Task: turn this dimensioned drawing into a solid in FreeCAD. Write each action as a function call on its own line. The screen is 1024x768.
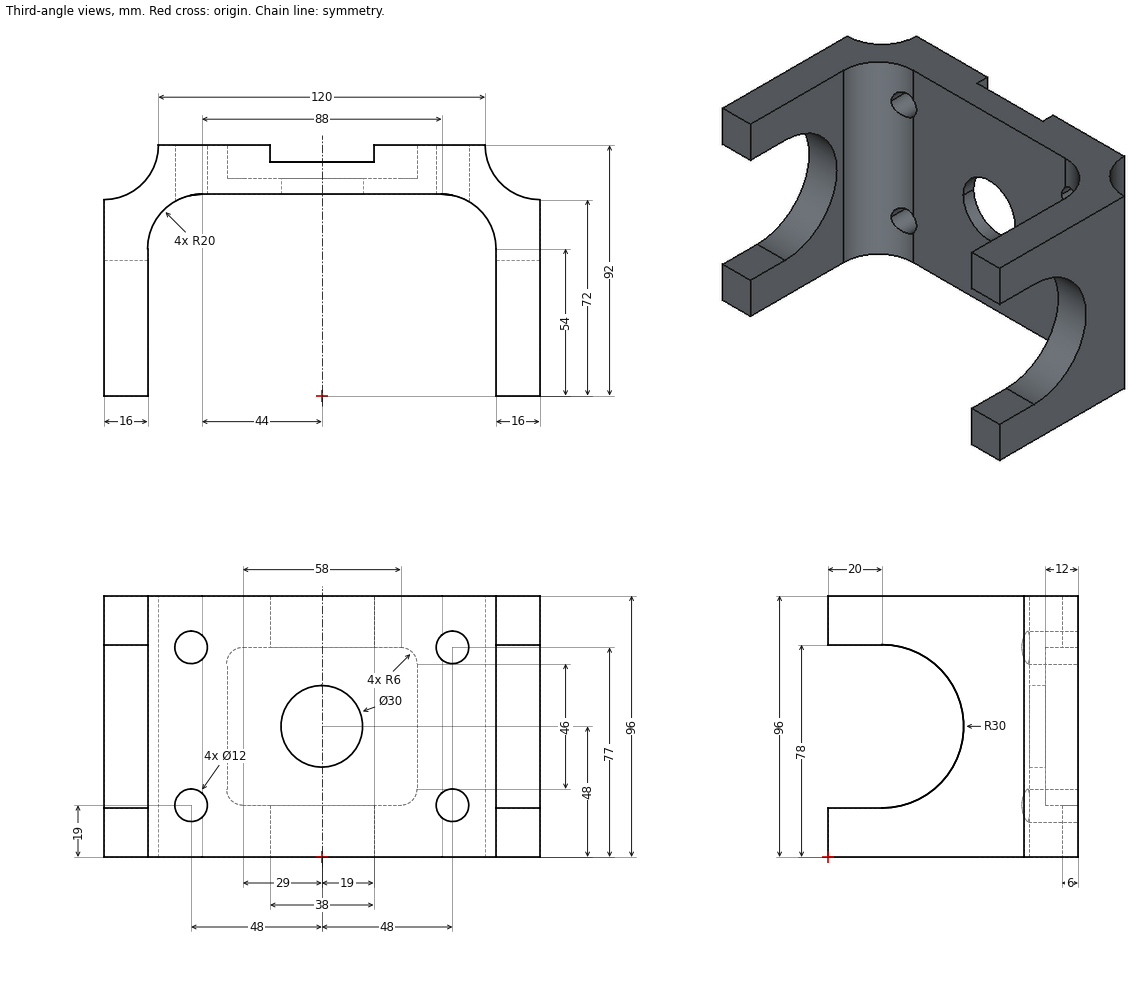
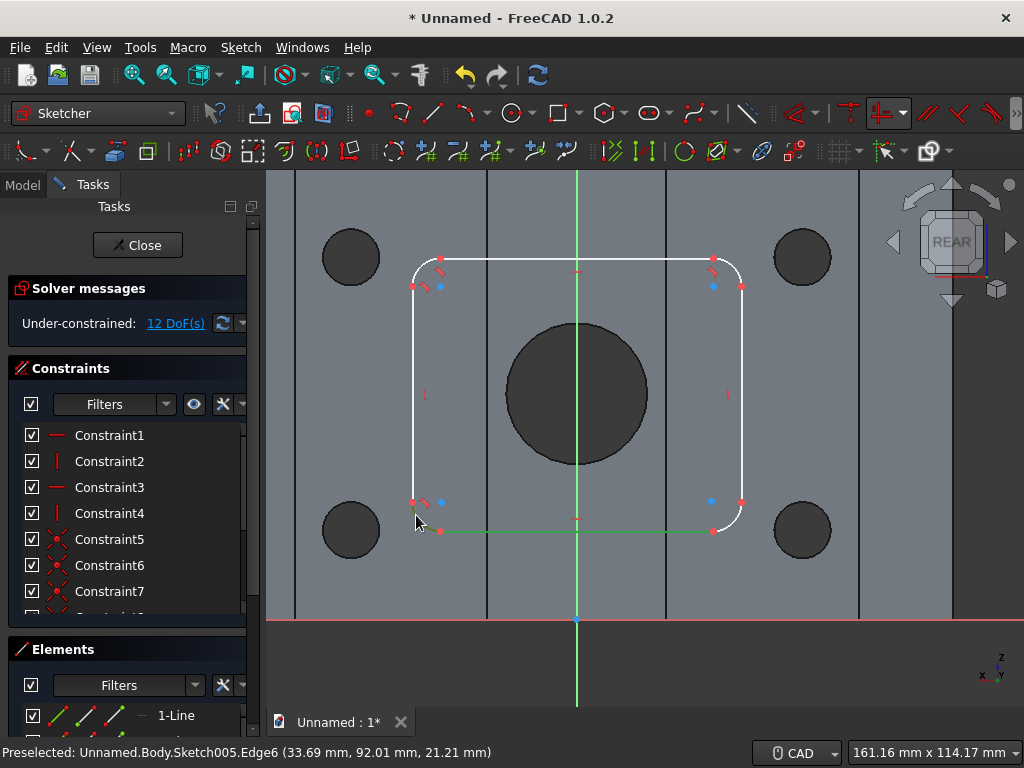
click(992, 114)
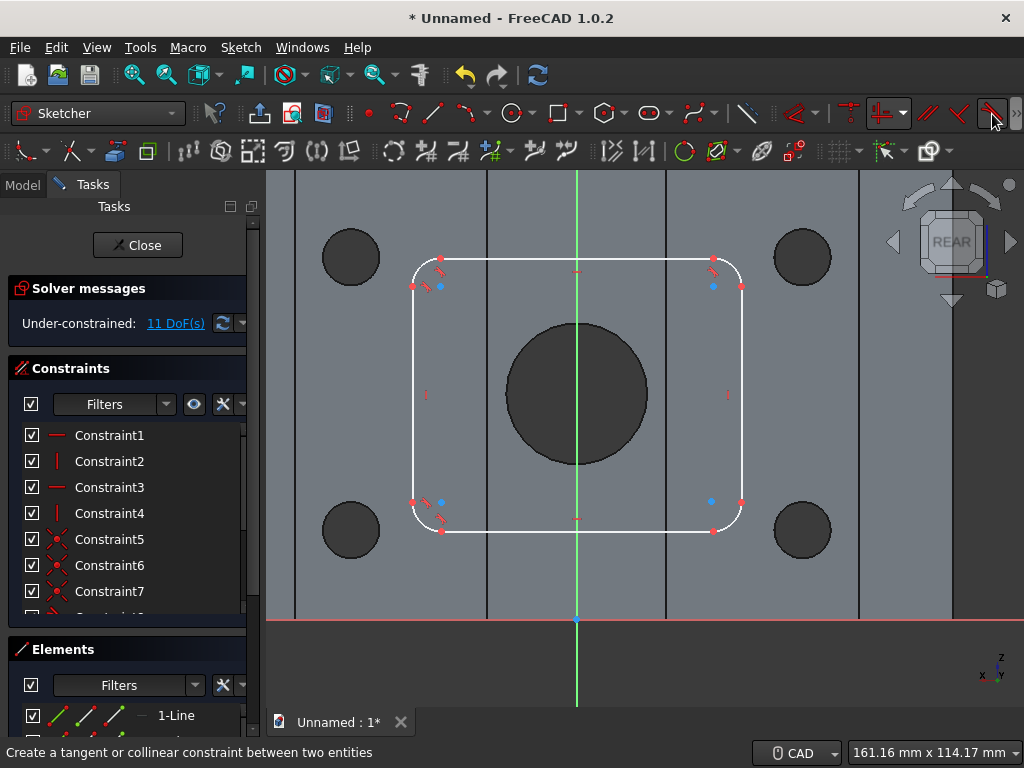
click(523, 532)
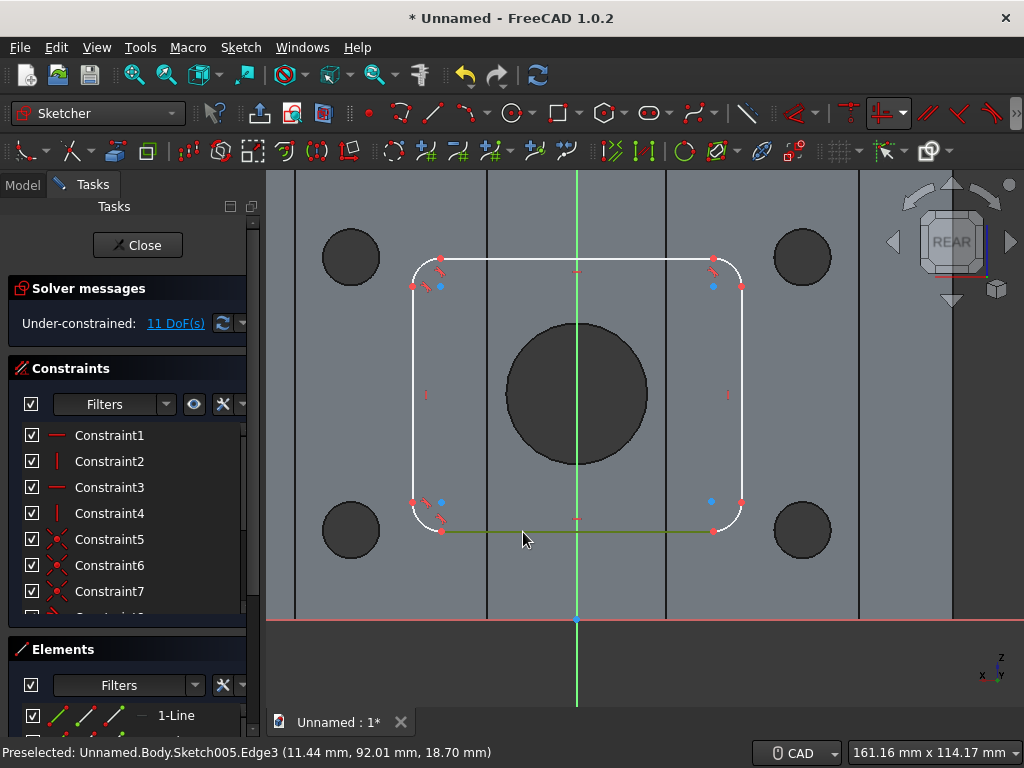
click(726, 528)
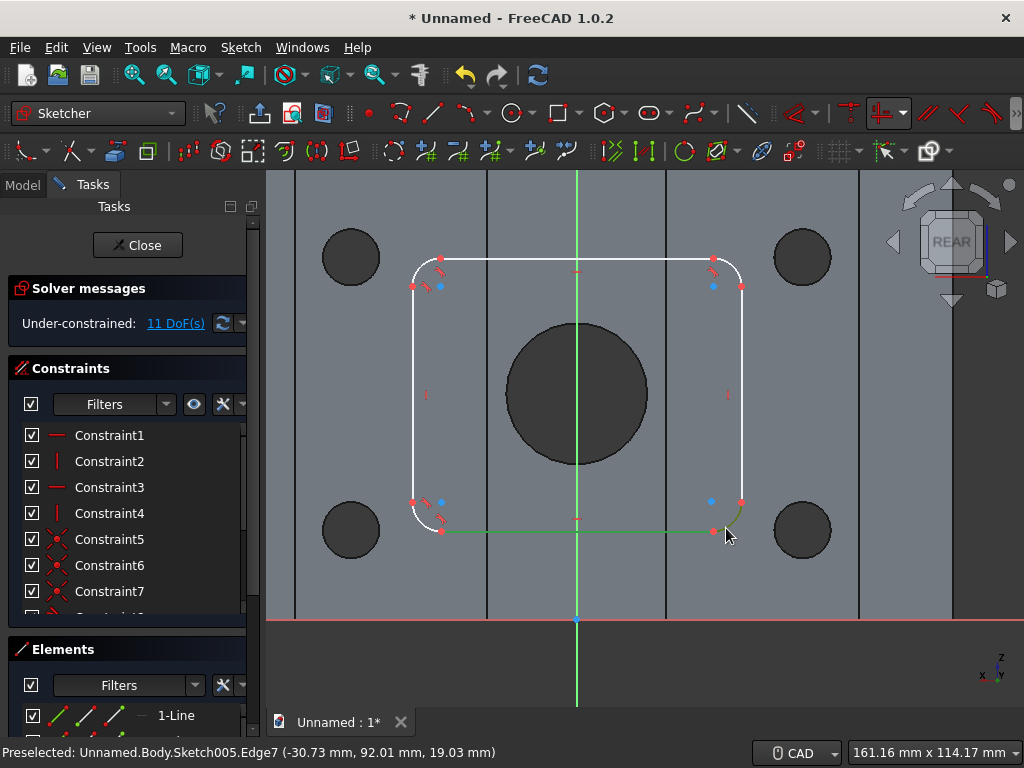
click(992, 114)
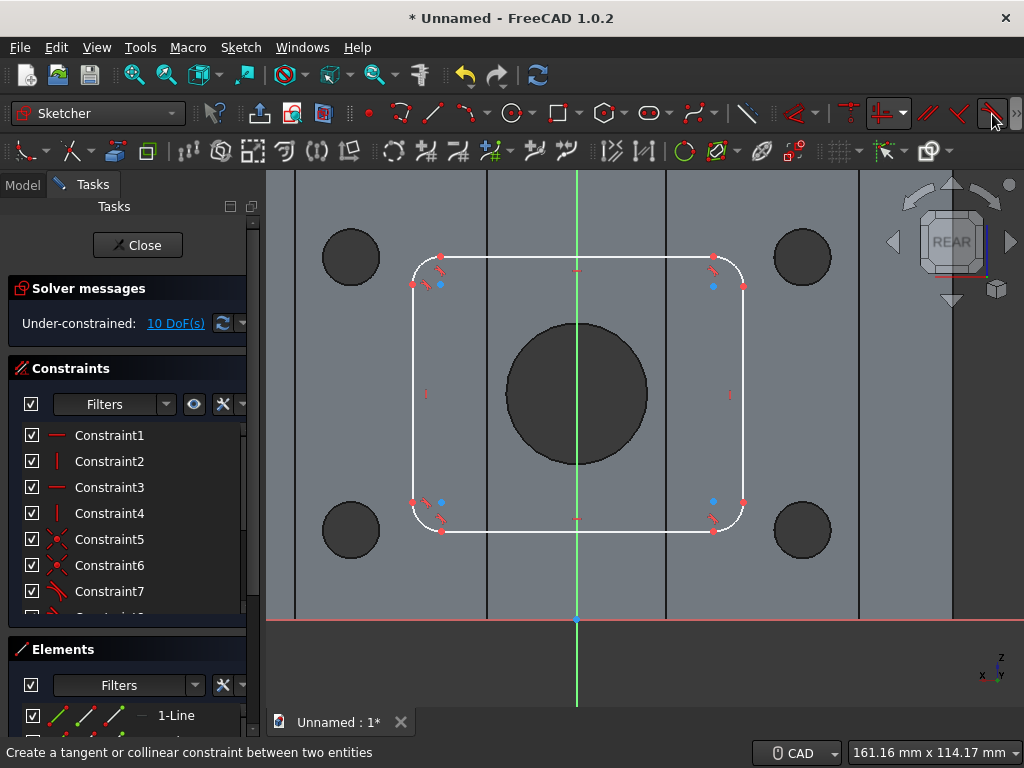
click(743, 438)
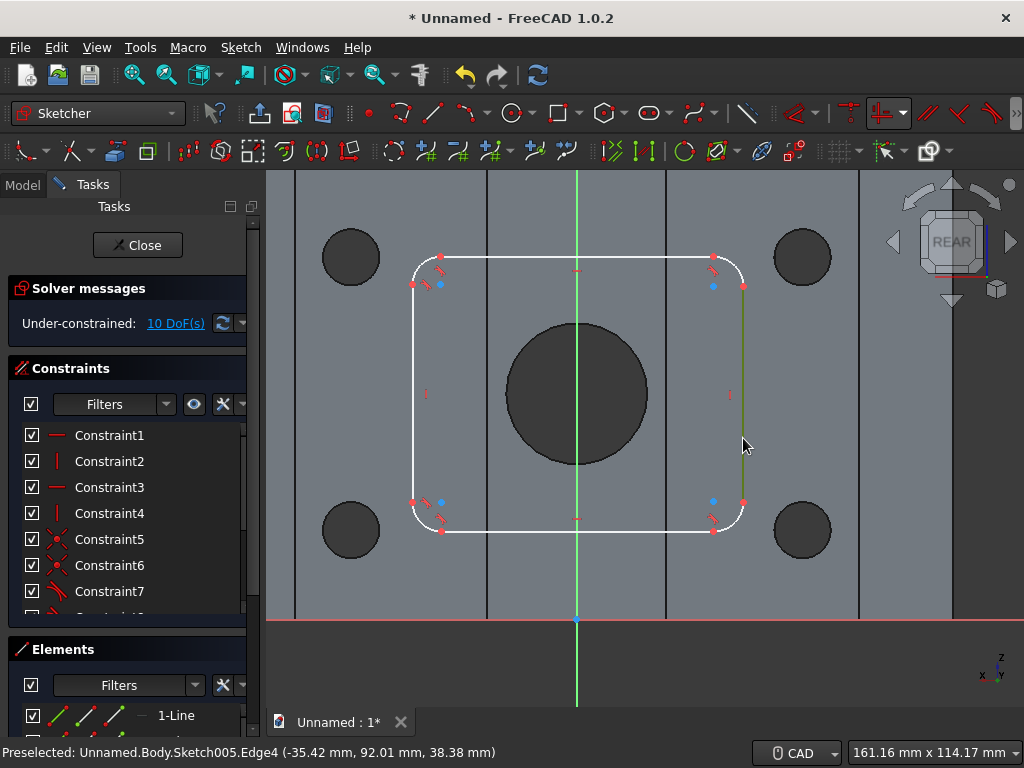
click(727, 528)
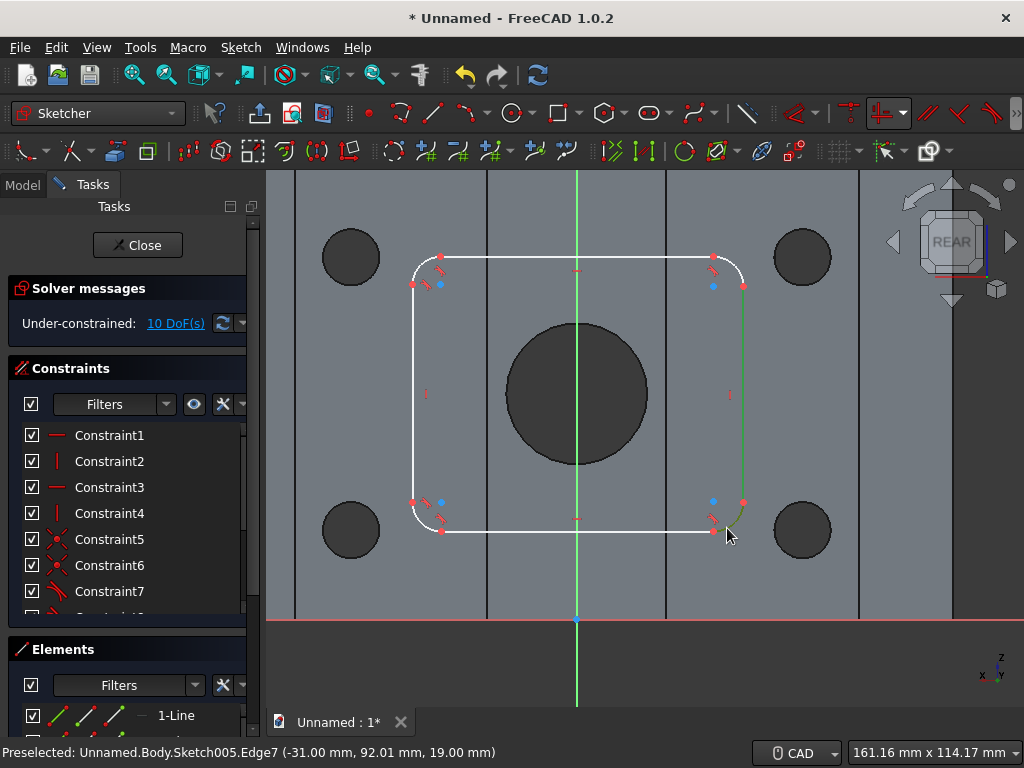
click(992, 114)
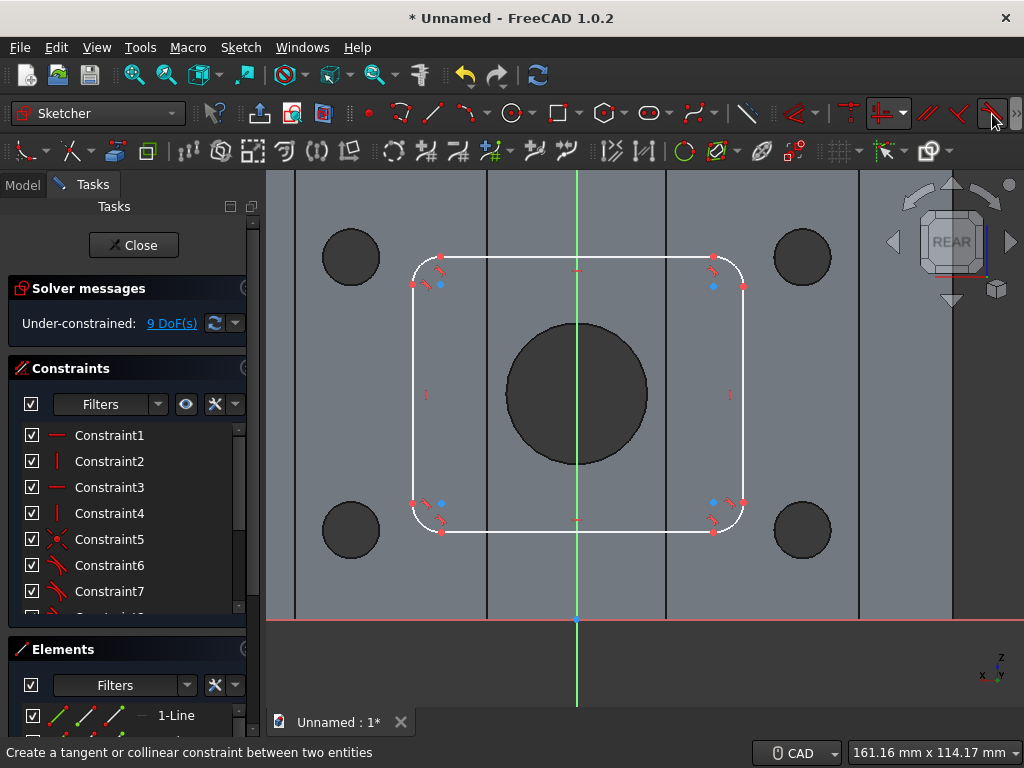
click(743, 438)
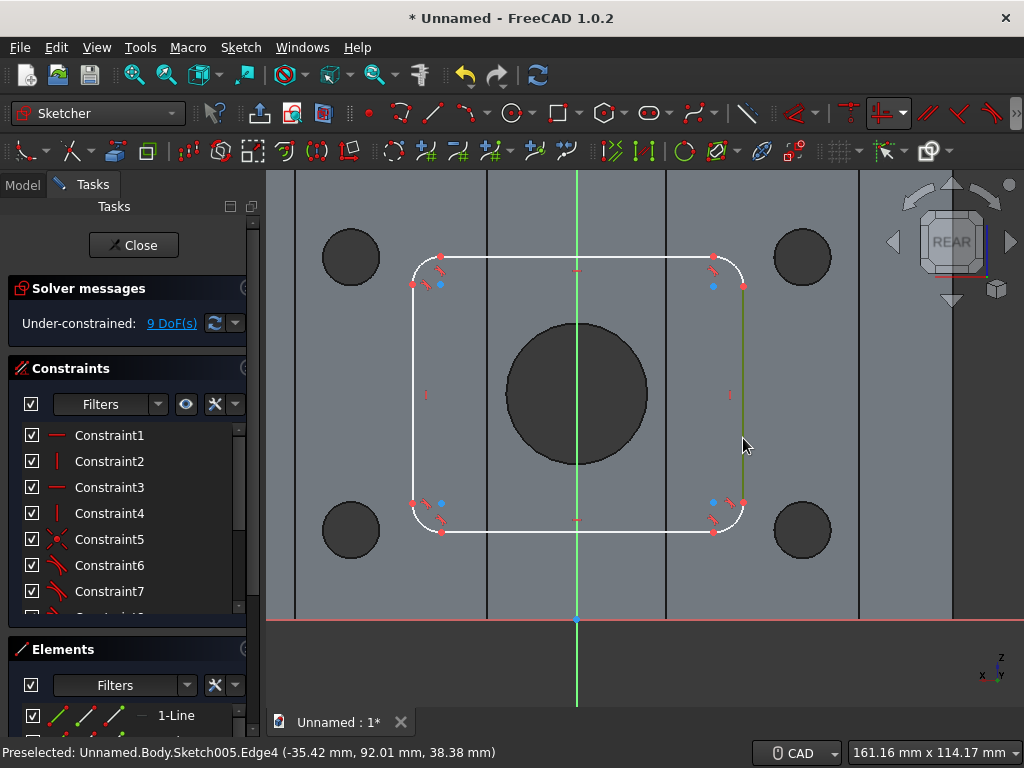
click(740, 273)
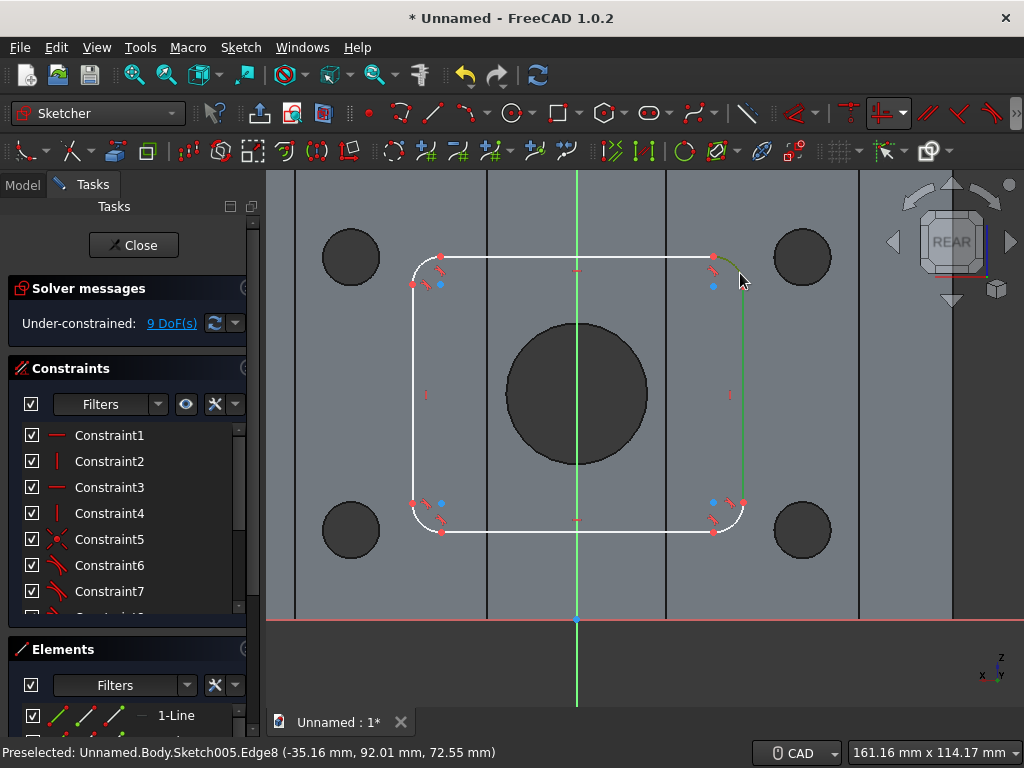
click(992, 114)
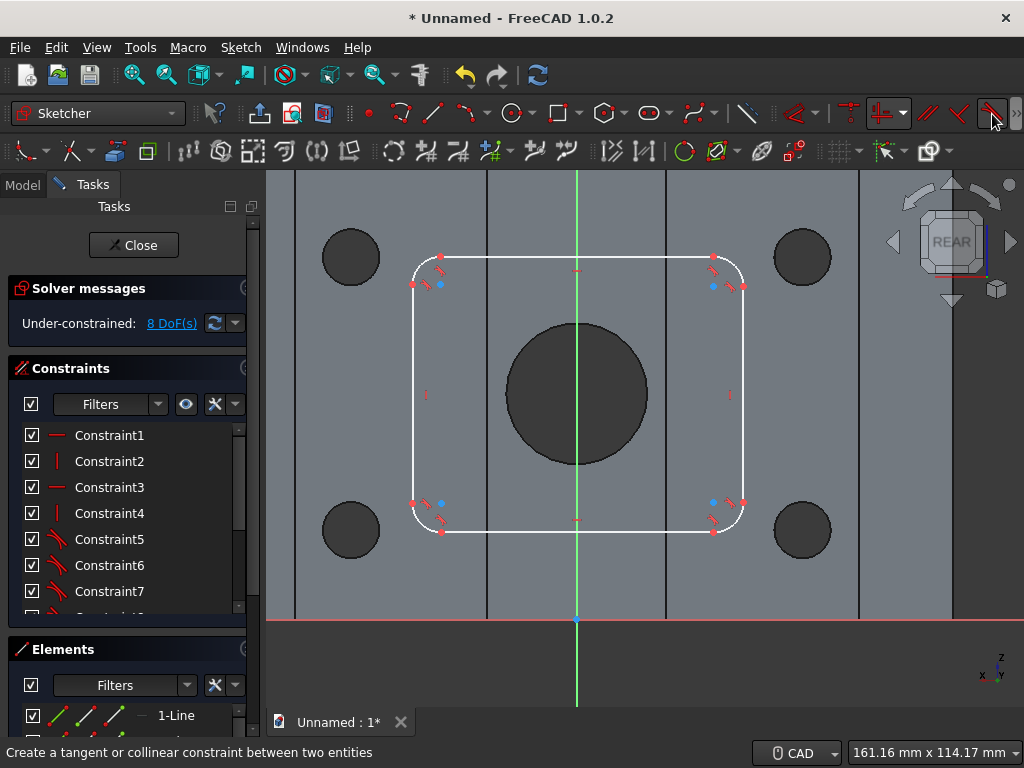
click(428, 260)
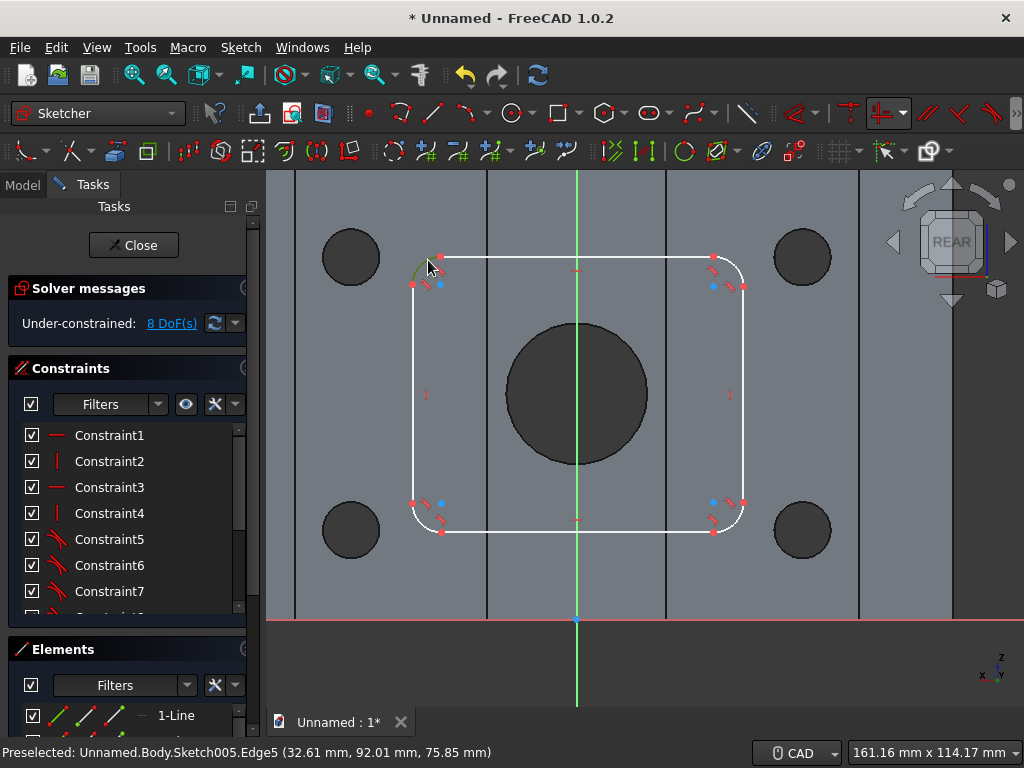
click(416, 516)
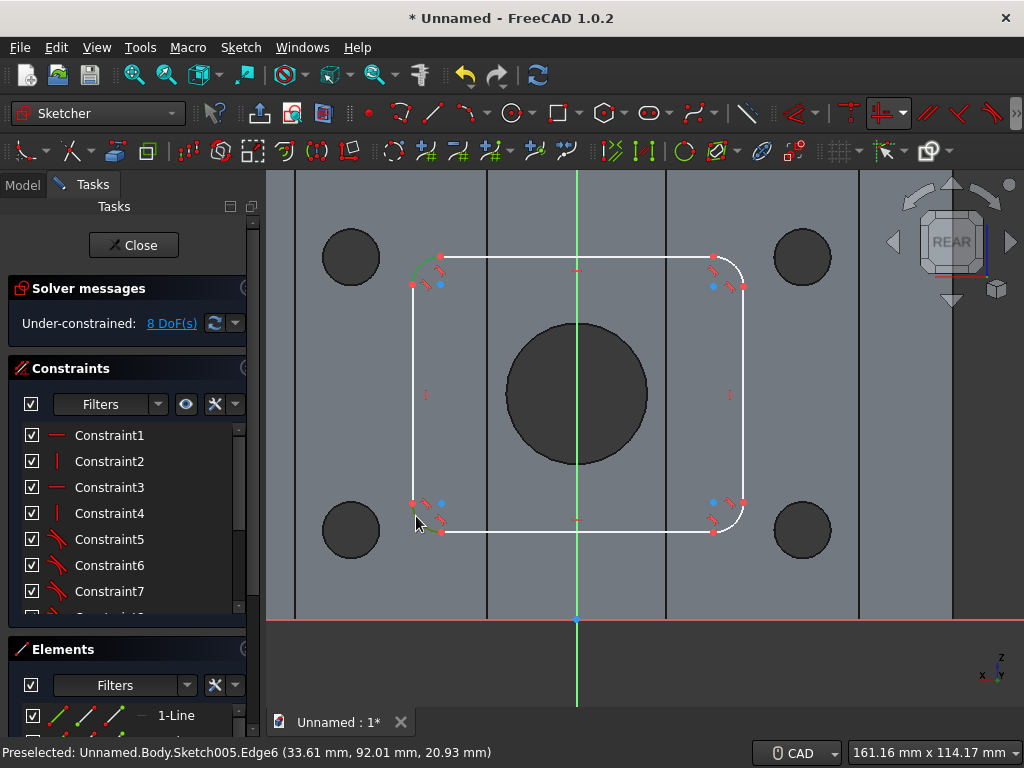
click(727, 529)